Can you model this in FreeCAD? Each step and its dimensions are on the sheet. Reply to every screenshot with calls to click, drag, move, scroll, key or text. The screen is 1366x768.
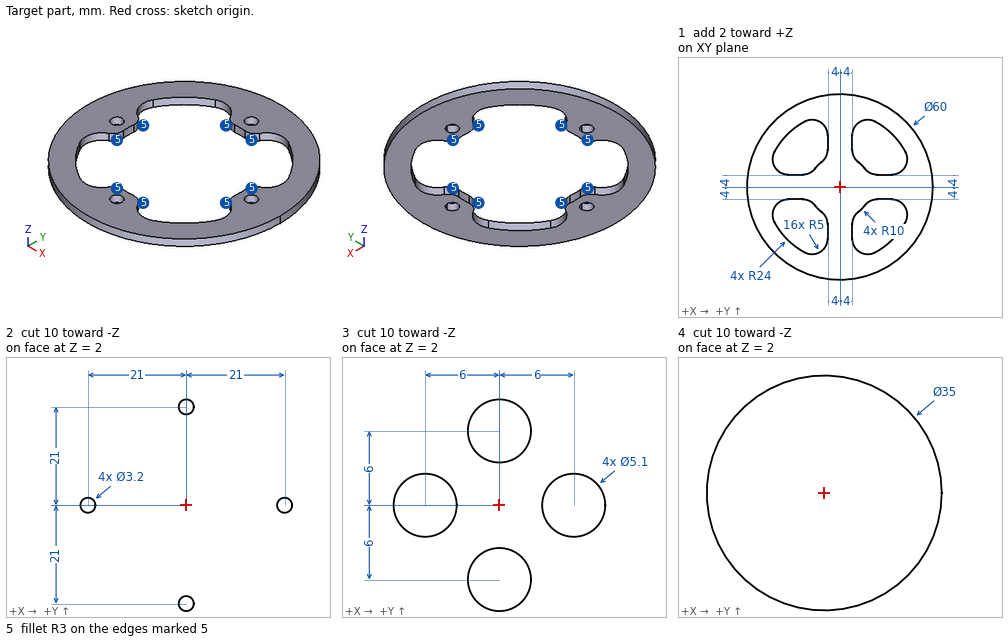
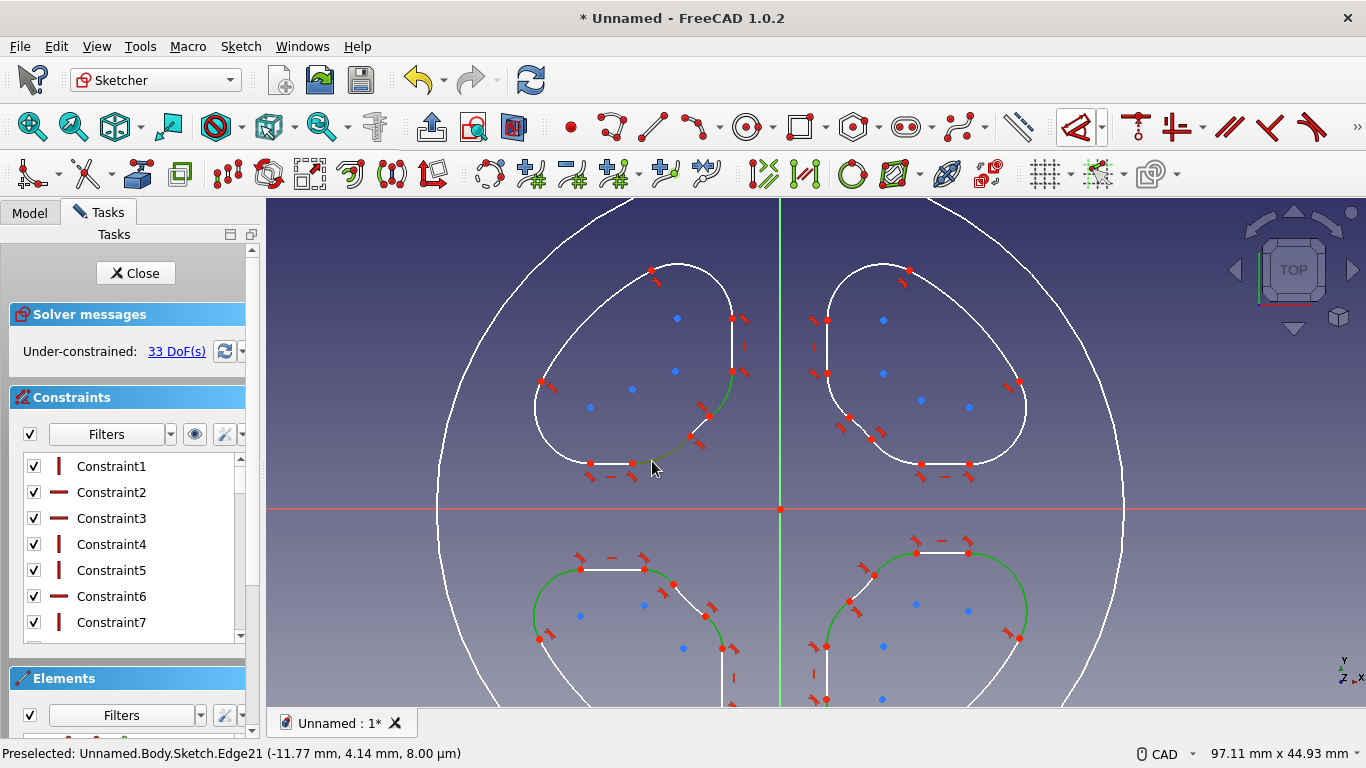
click(535, 415)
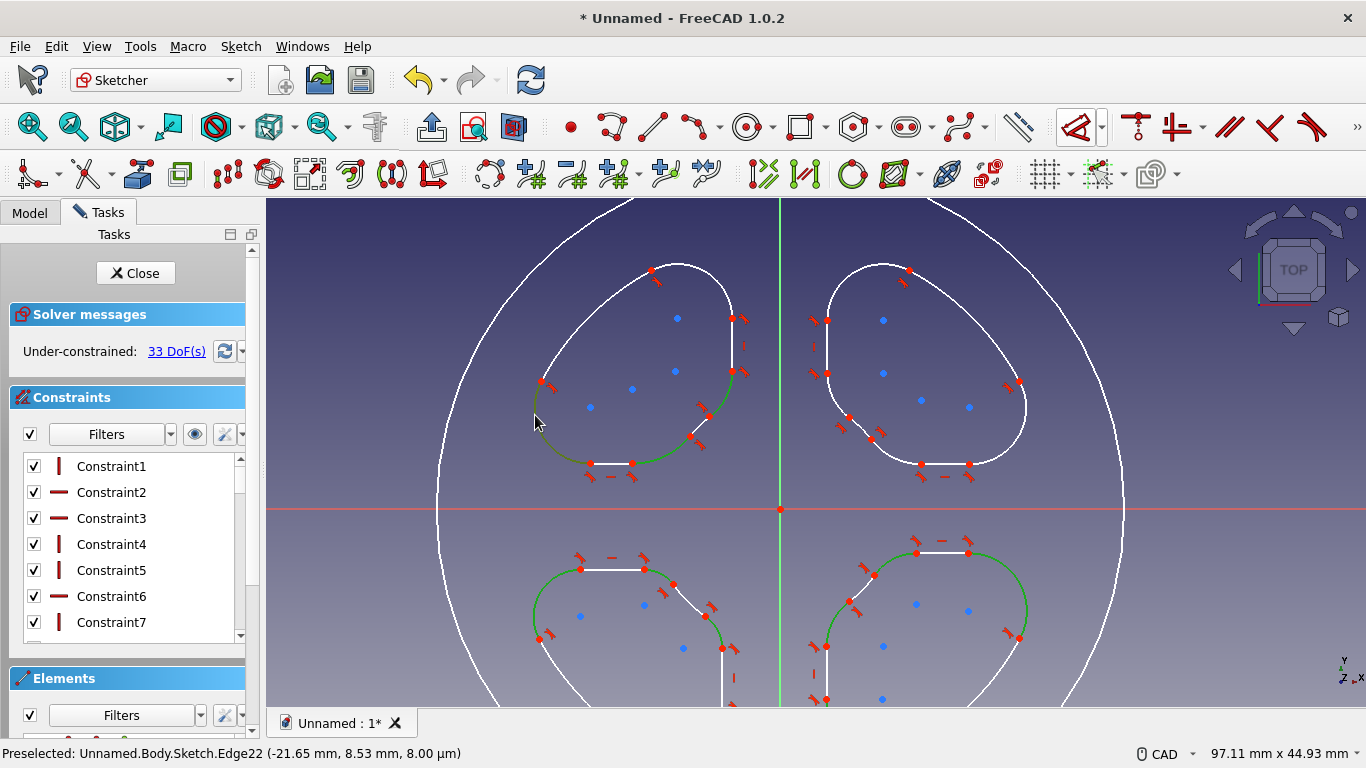
click(722, 287)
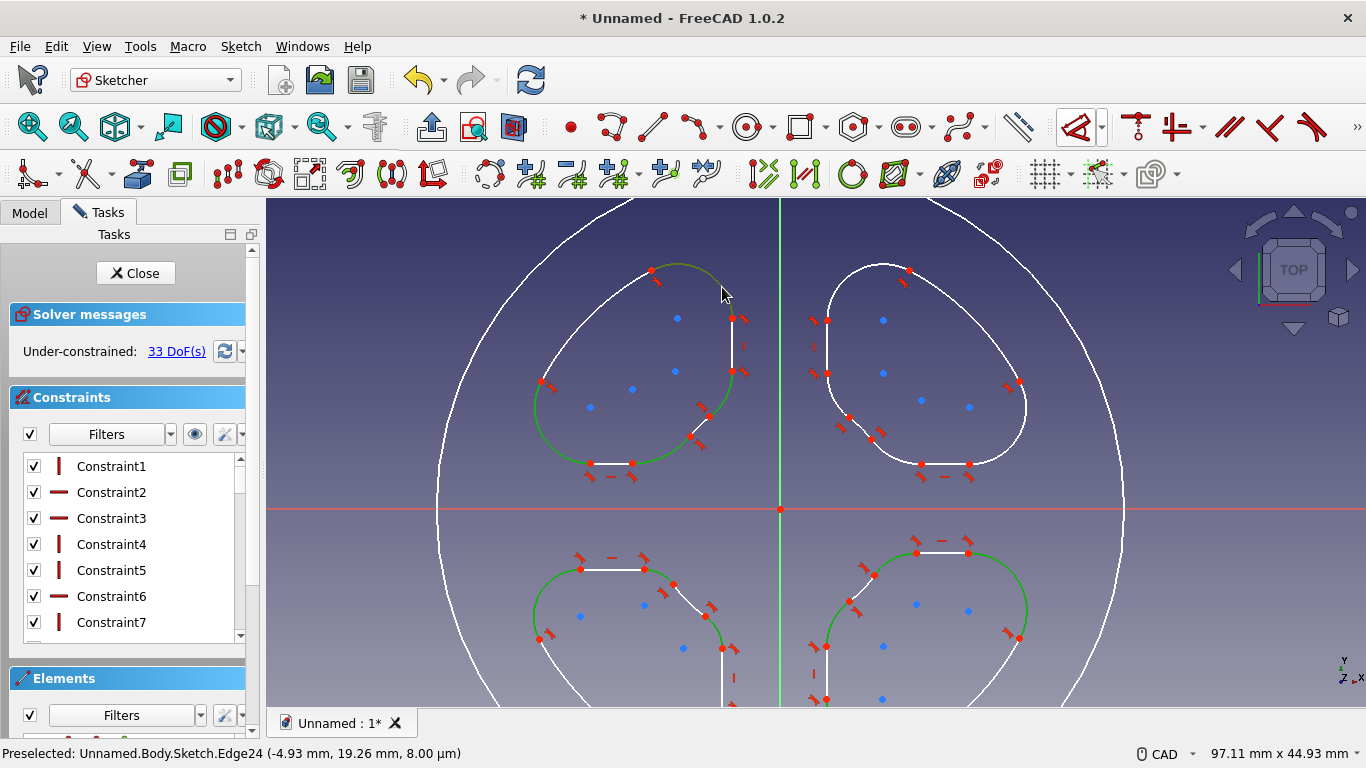
click(877, 265)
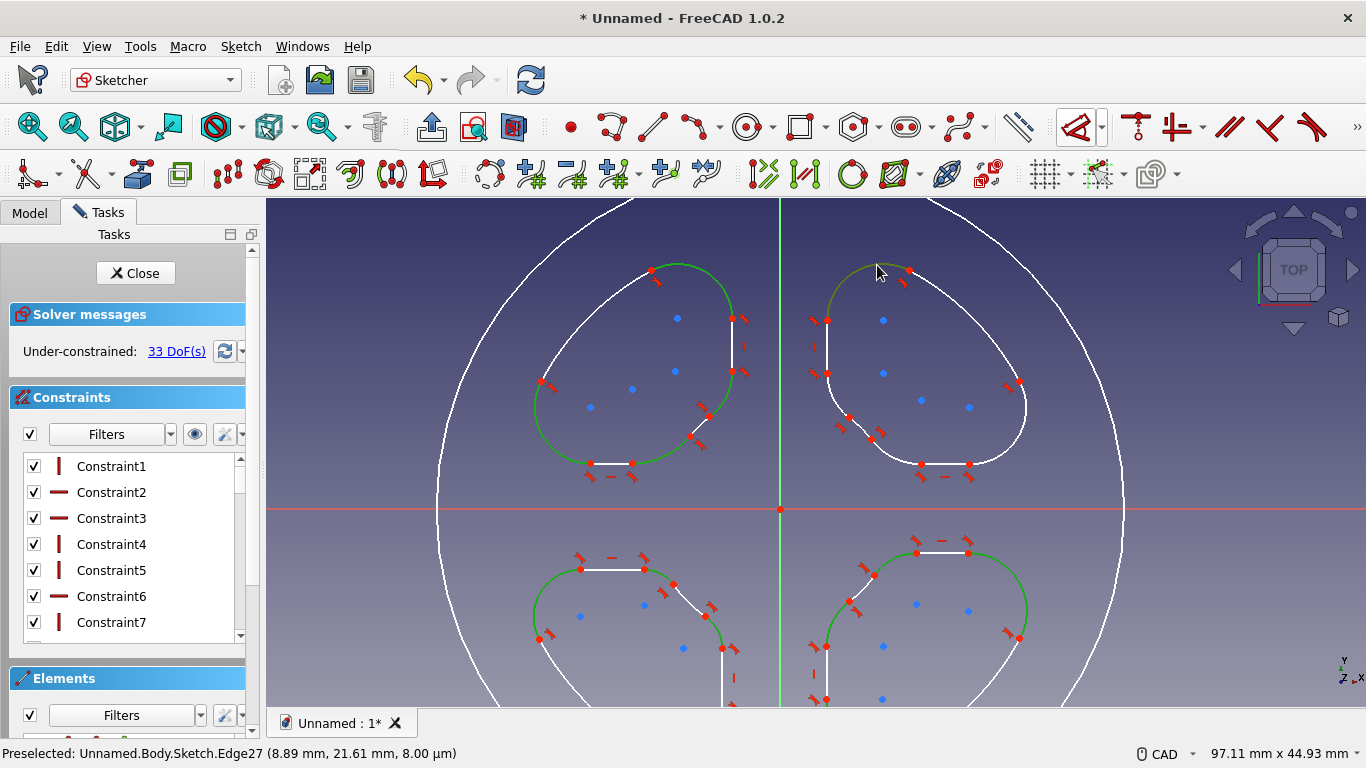
click(1002, 454)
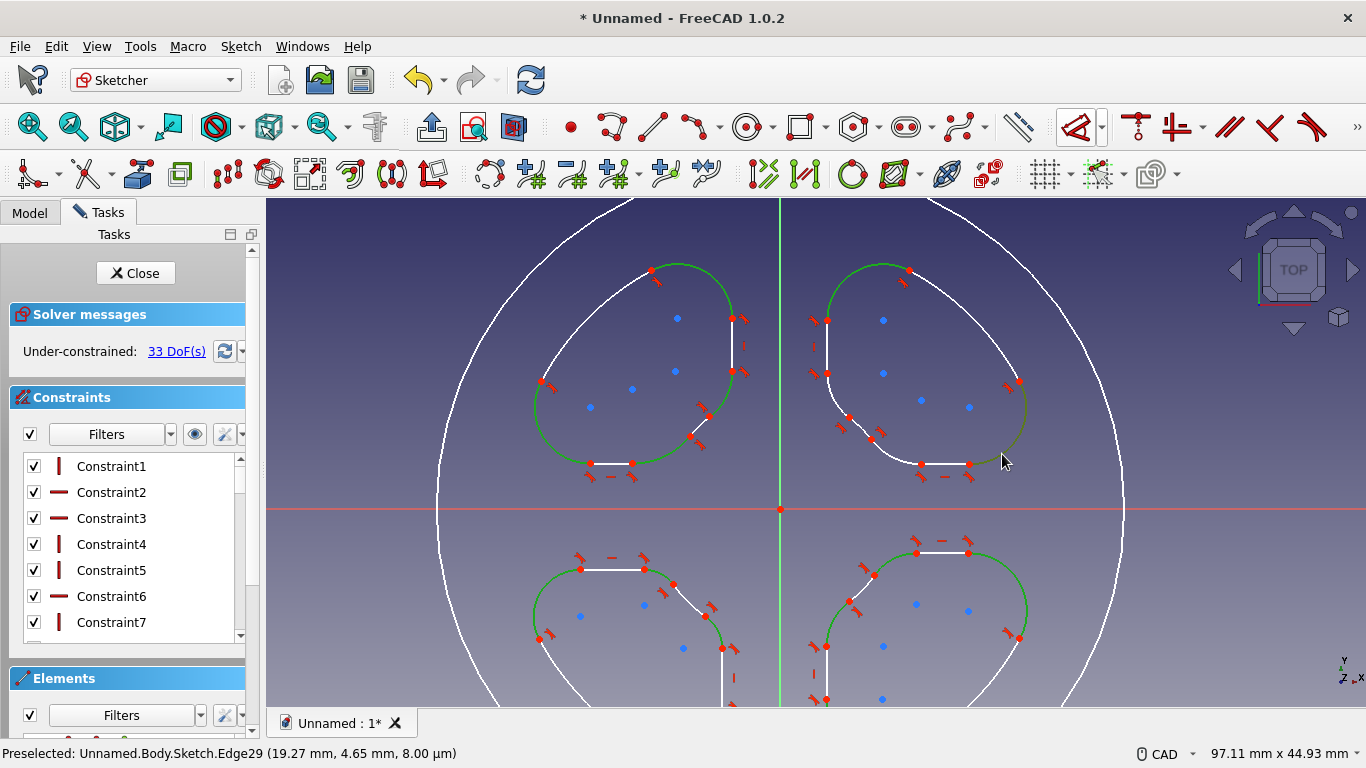
click(884, 452)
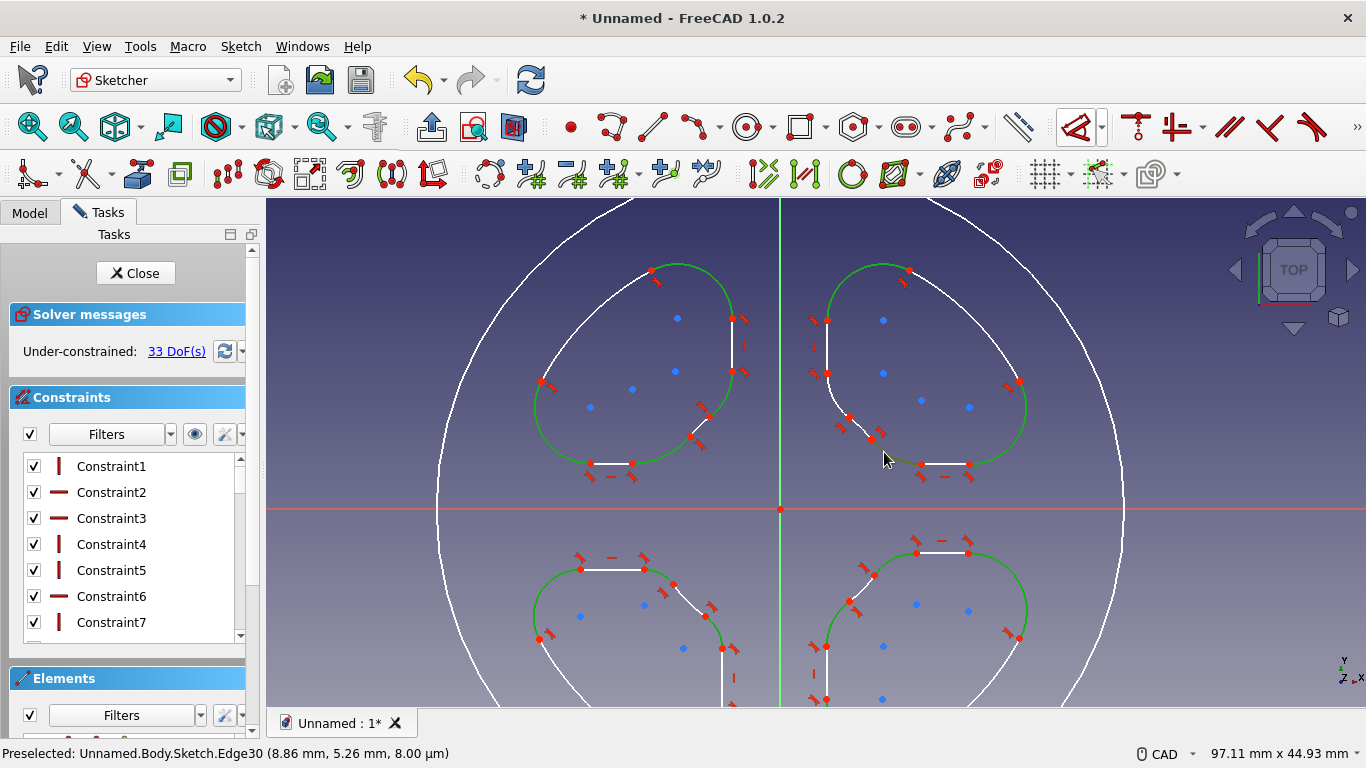
click(830, 389)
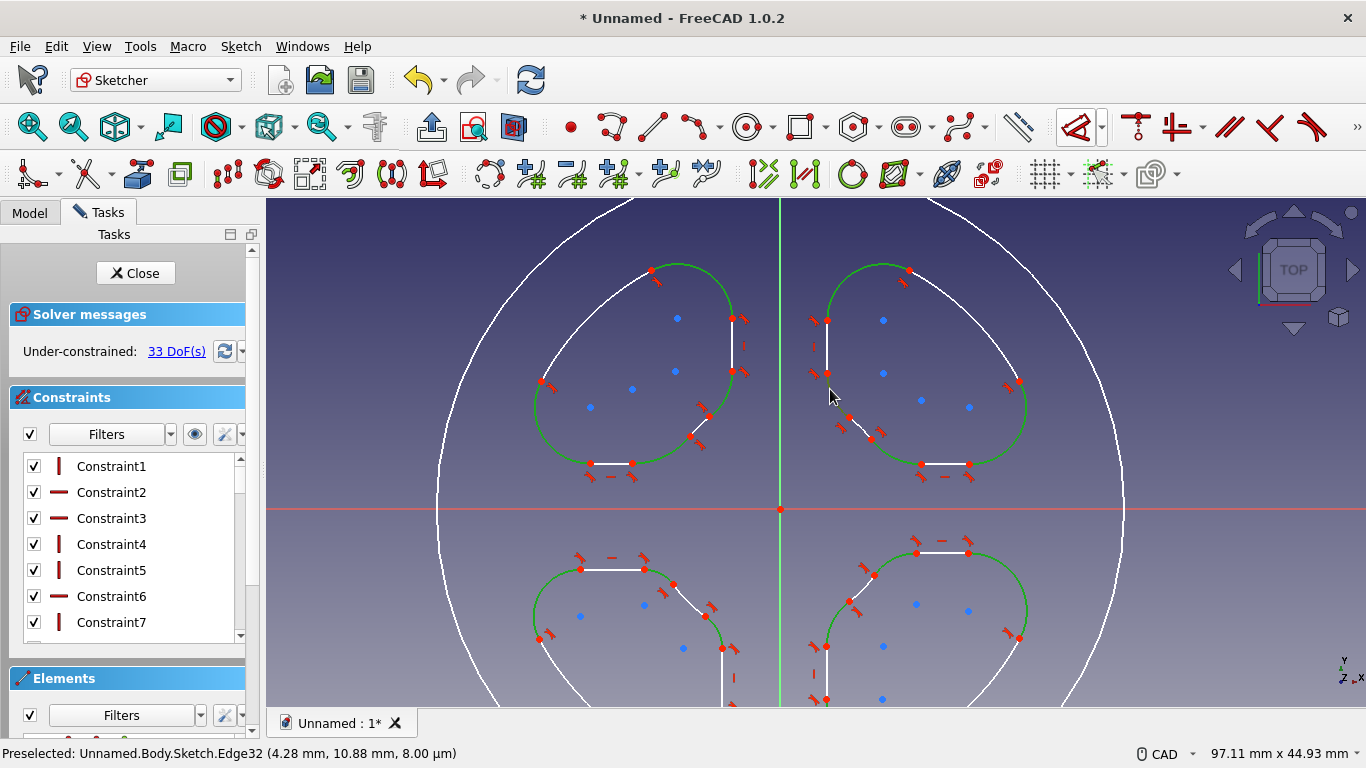
key(e)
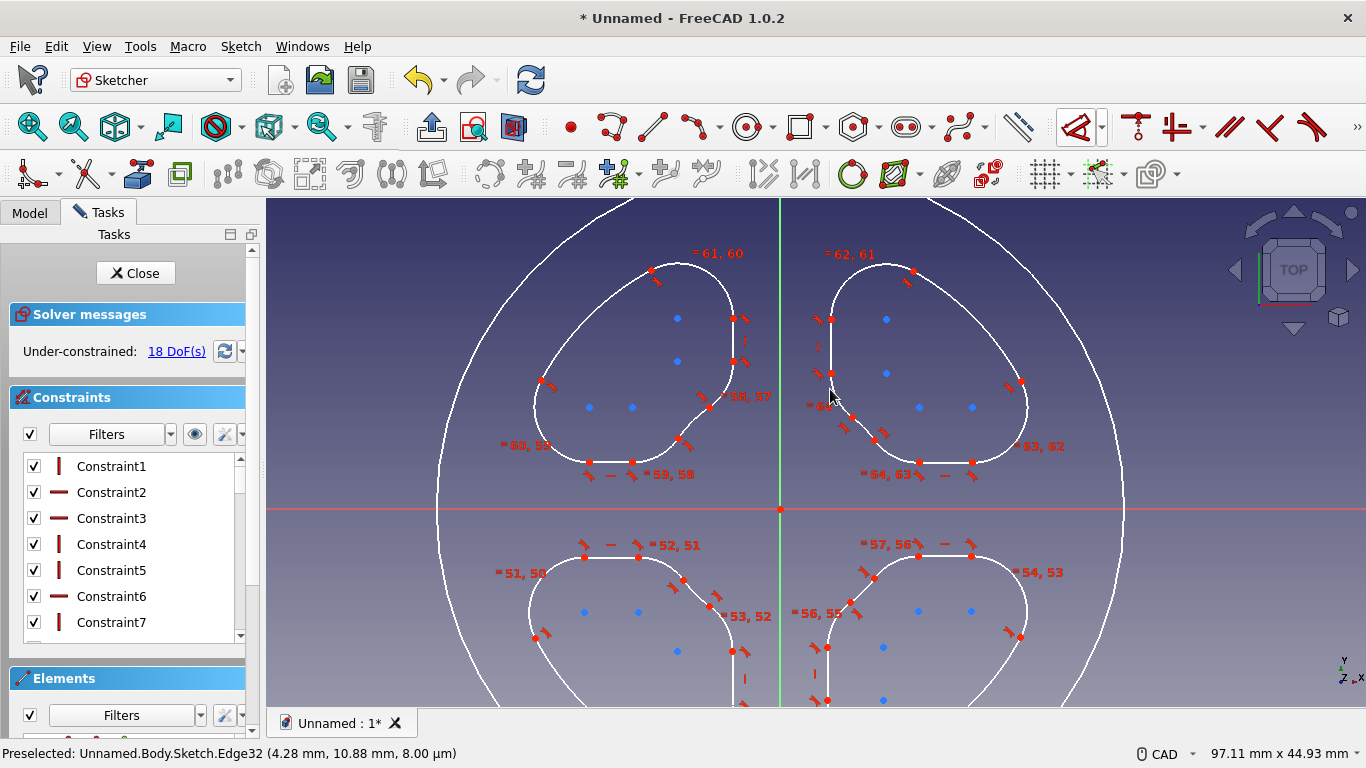
click(553, 667)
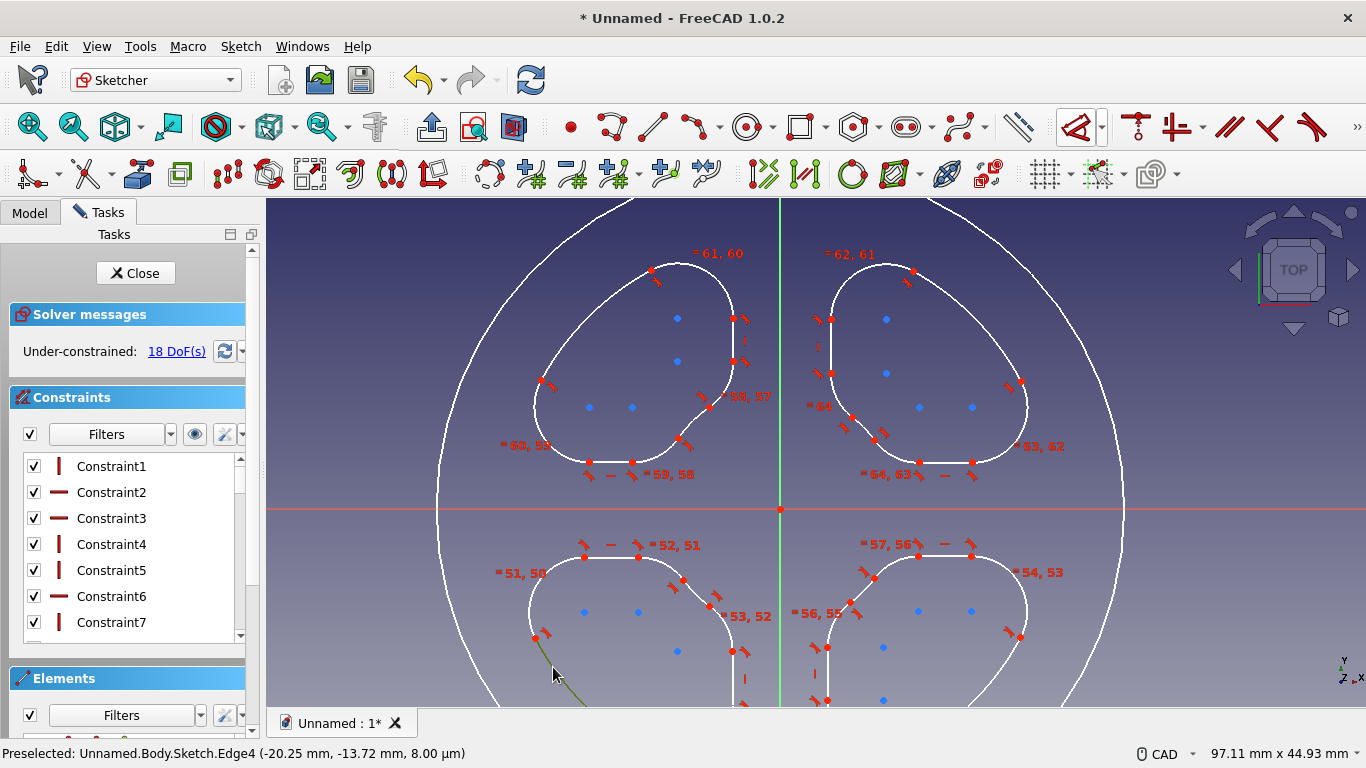
click(994, 678)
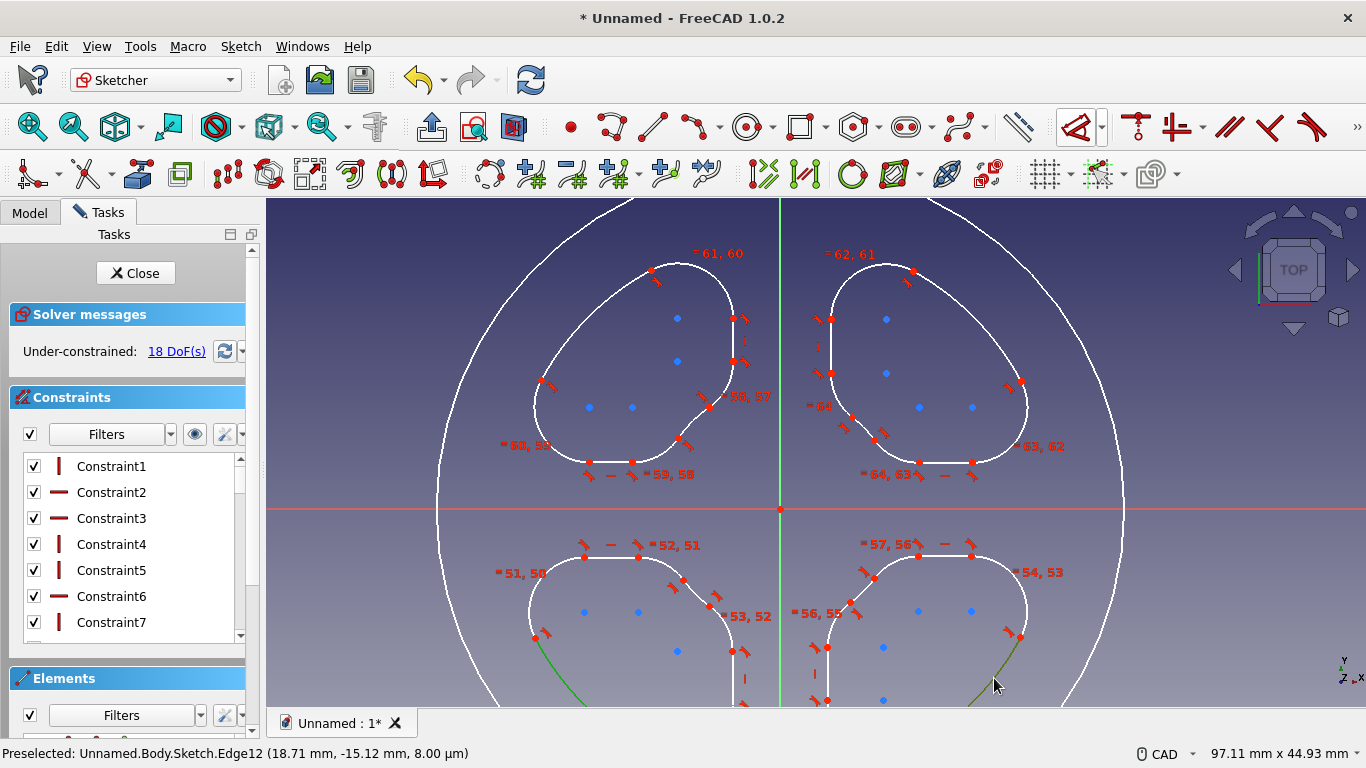
click(612, 296)